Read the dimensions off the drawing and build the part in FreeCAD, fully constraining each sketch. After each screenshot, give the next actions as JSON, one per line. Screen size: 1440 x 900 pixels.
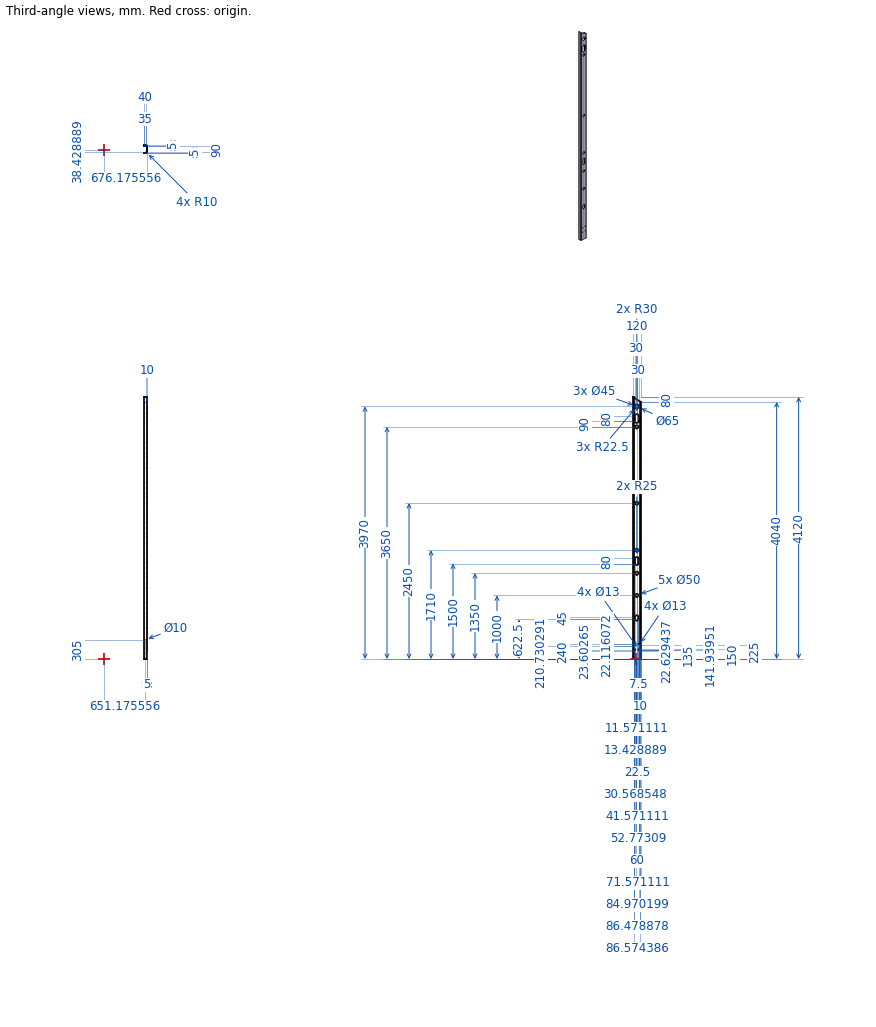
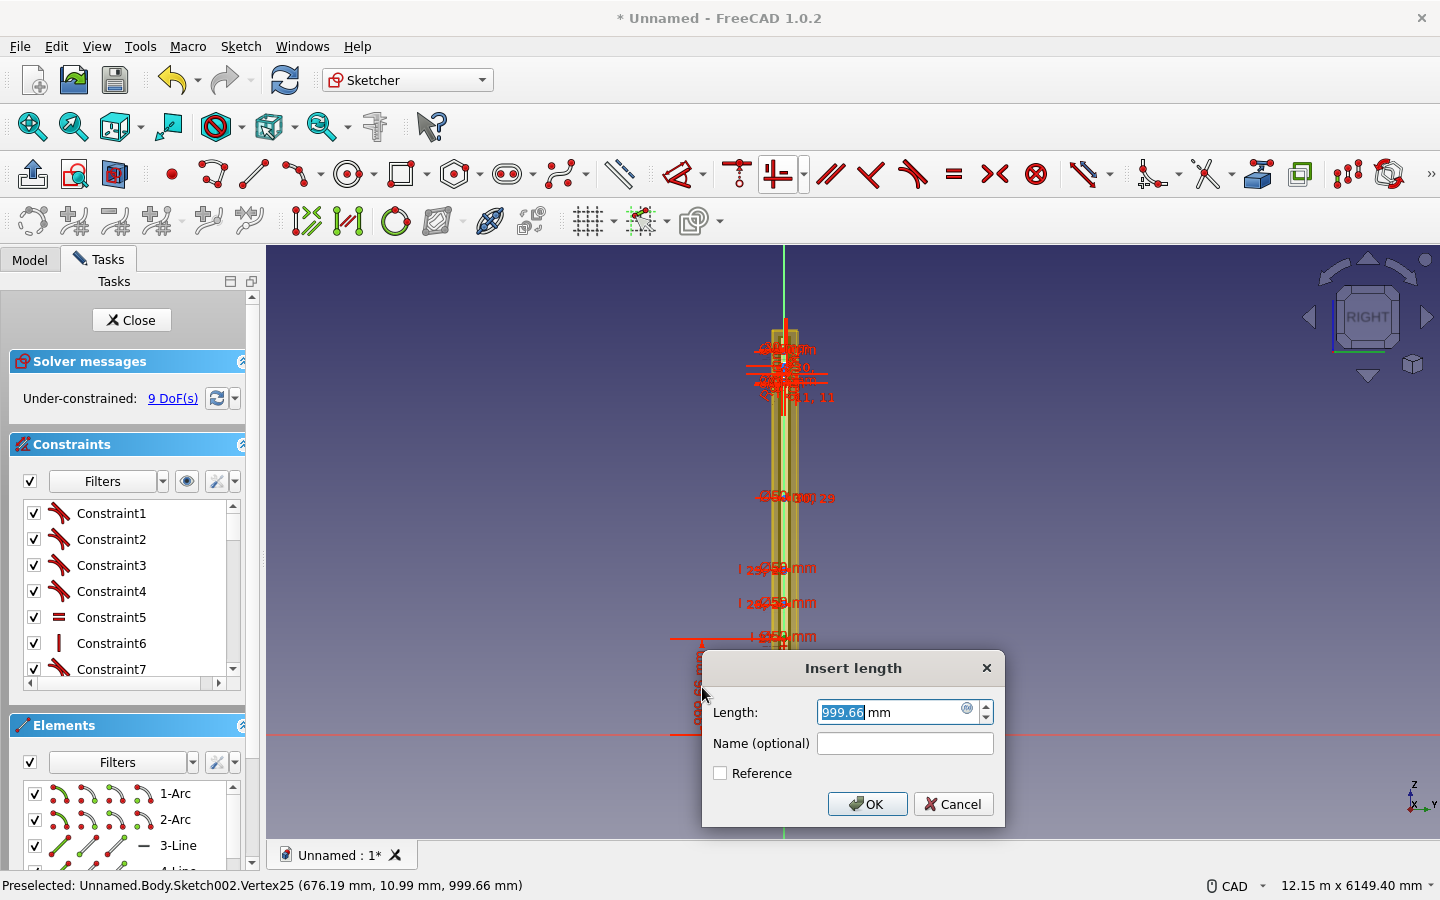
{"action": "type", "text": "1000"}
{"action": "key", "text": "Return"}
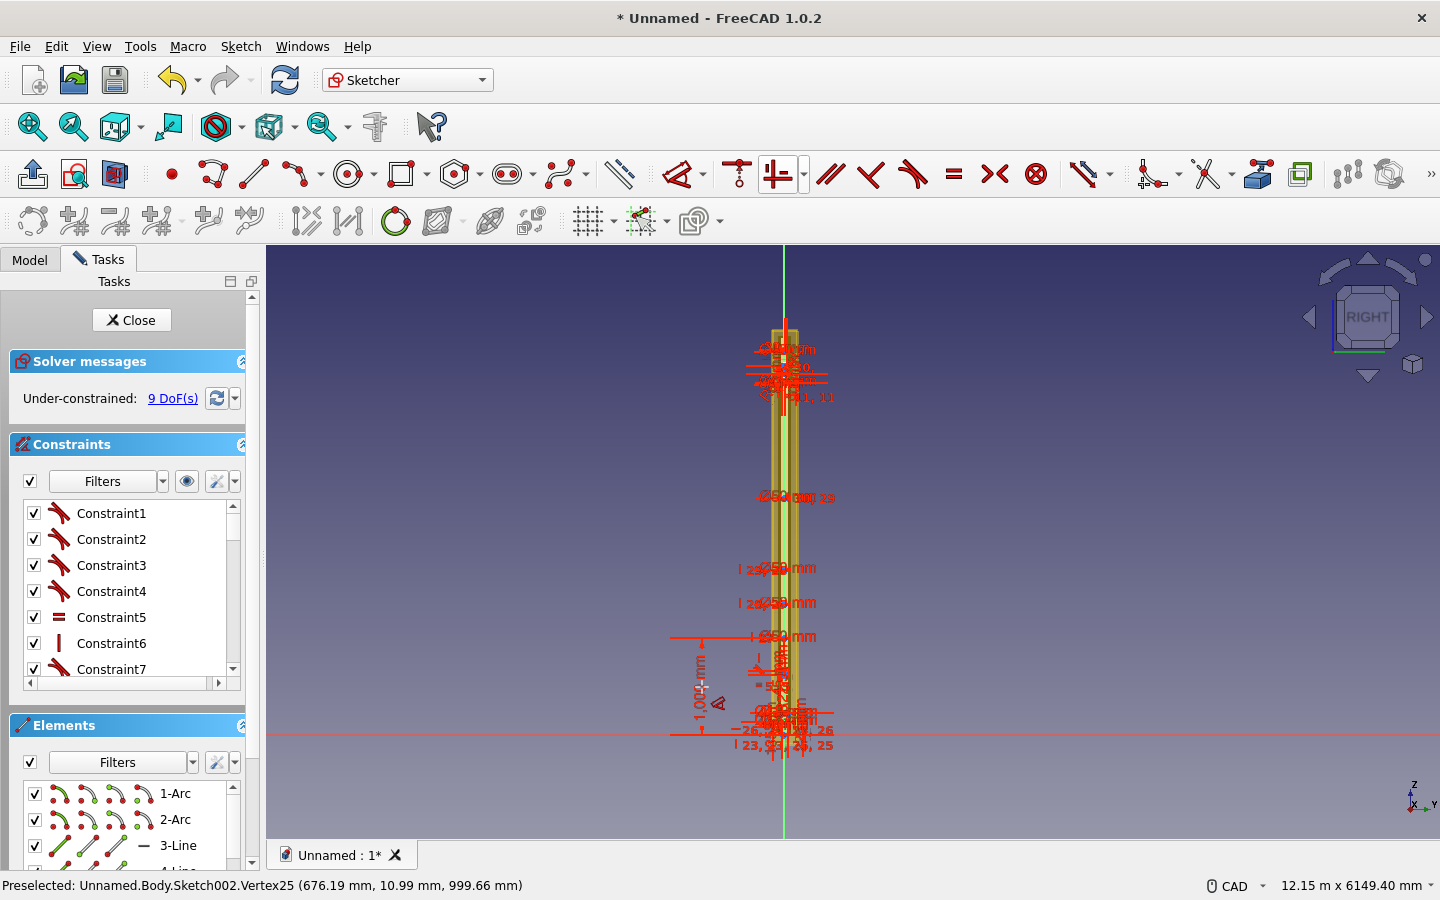
{"action": "left_click", "coordinate": [785, 605]}
{"action": "left_click", "coordinate": [750, 640]}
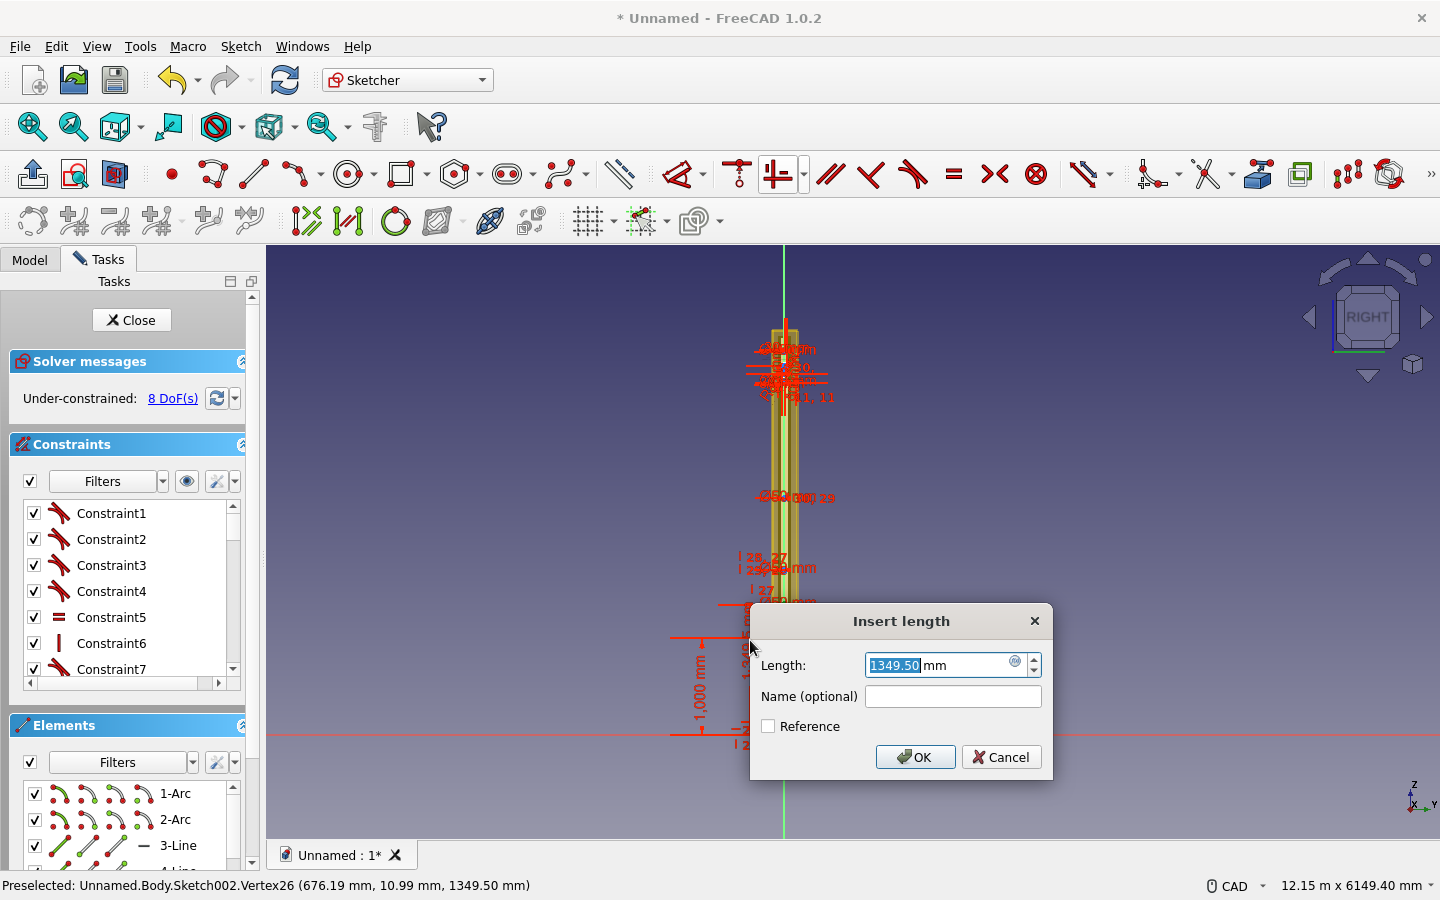
{"action": "type", "text": "1350"}
{"action": "key", "text": "Return"}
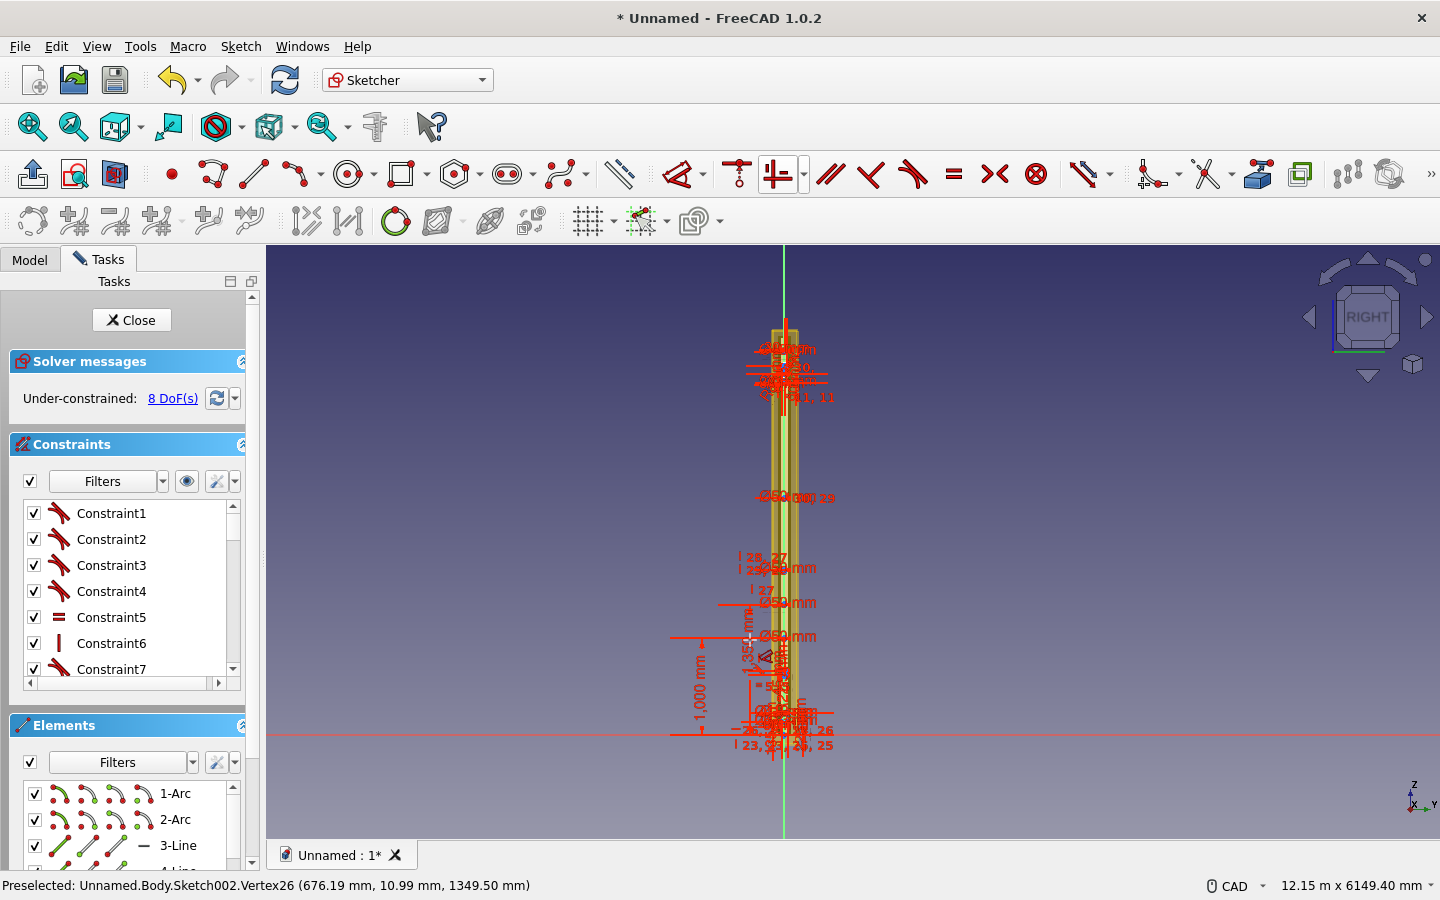
{"action": "left_click", "coordinate": [785, 352]}
{"action": "left_click", "coordinate": [750, 543]}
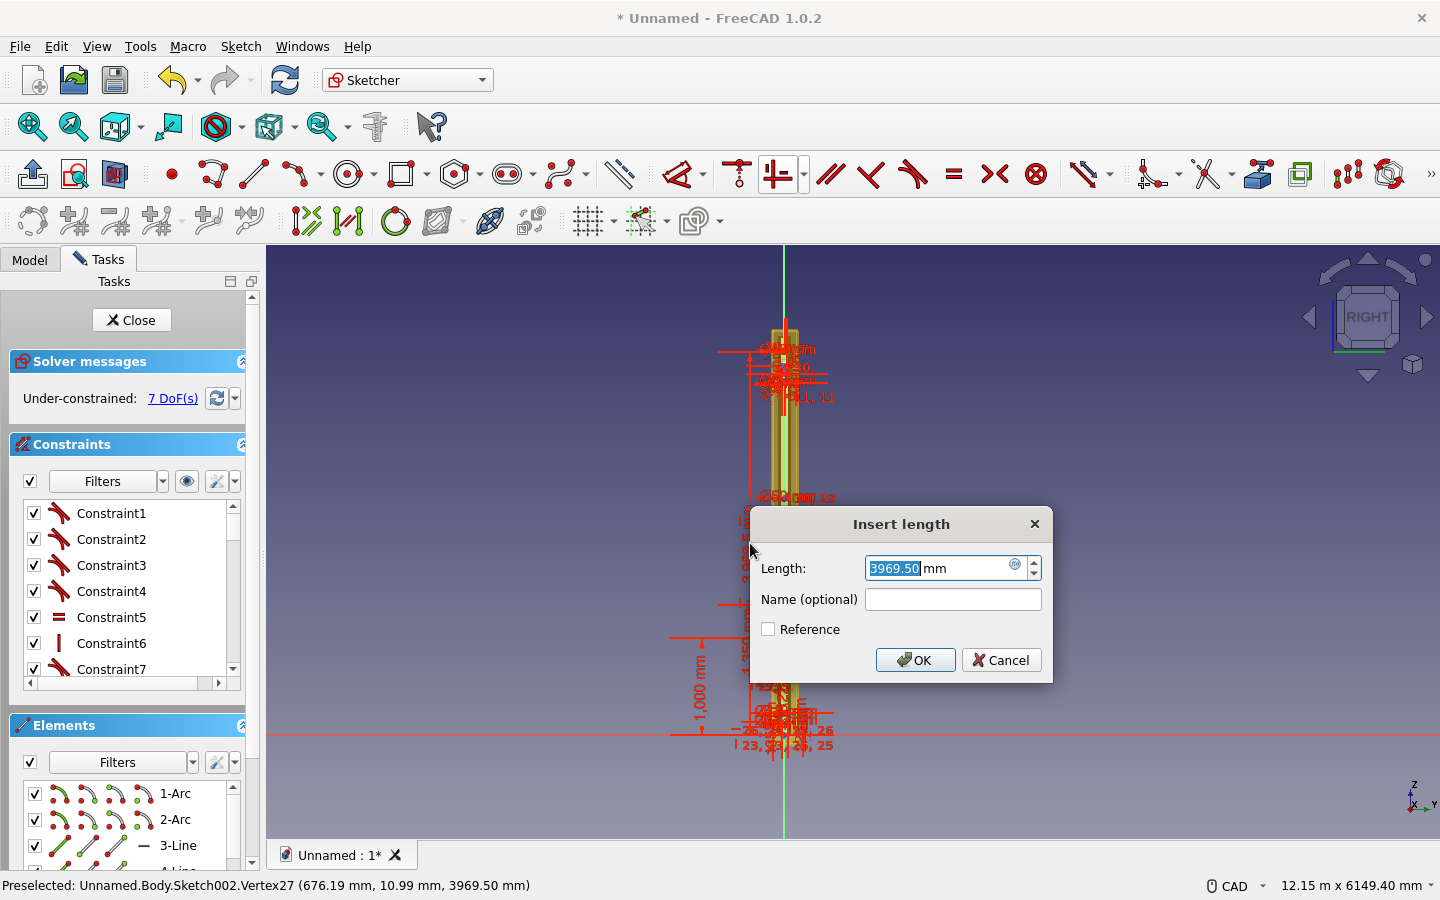
{"action": "type", "text": "3970"}
{"action": "key", "text": "Return"}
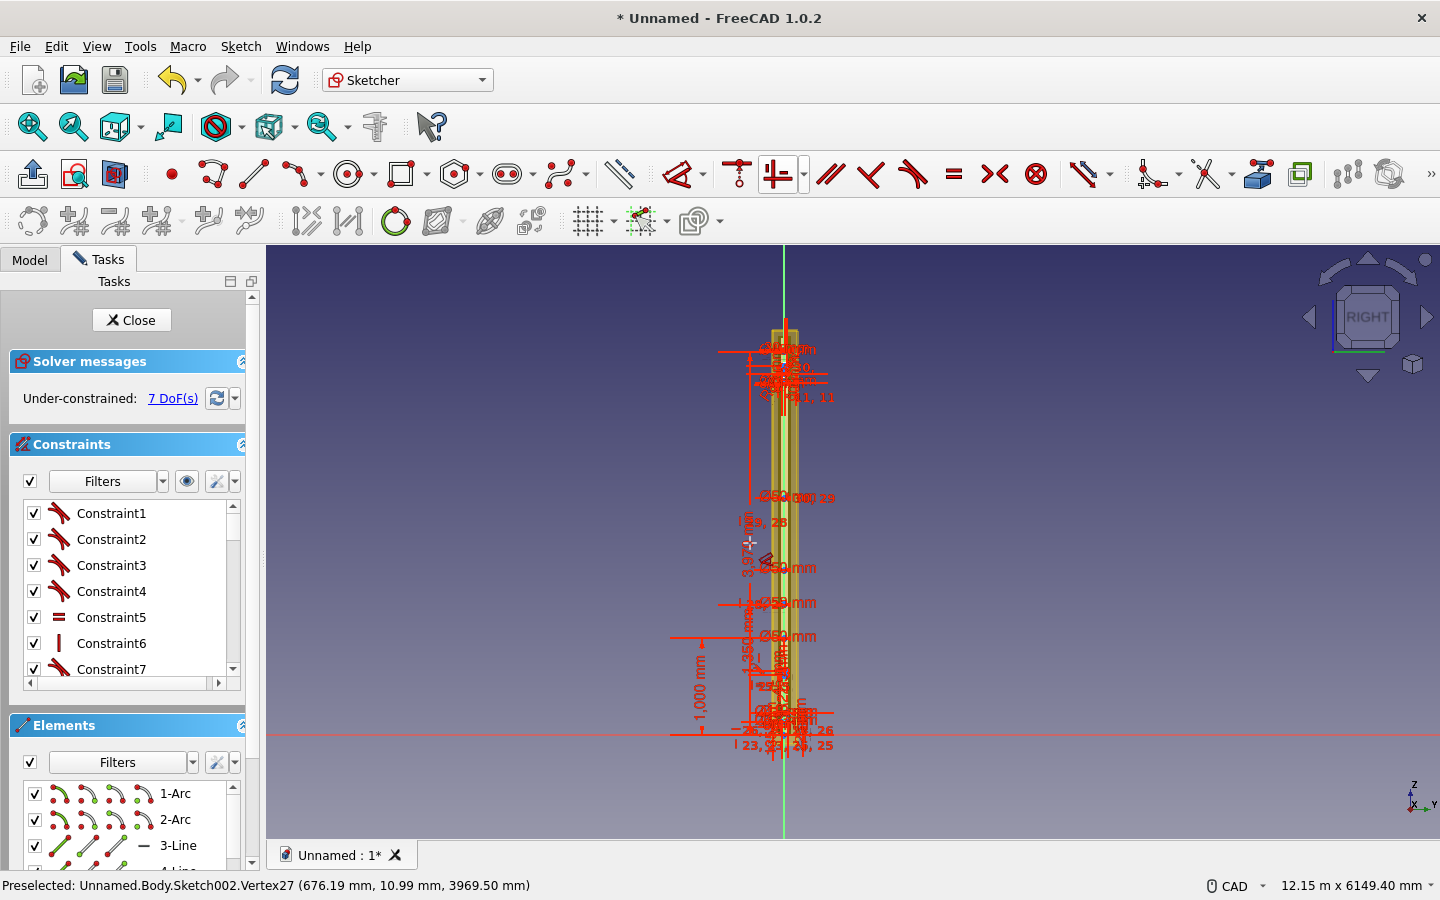
{"action": "scroll", "coordinate": [785, 383], "scroll_direction": "up", "scroll_amount": 2}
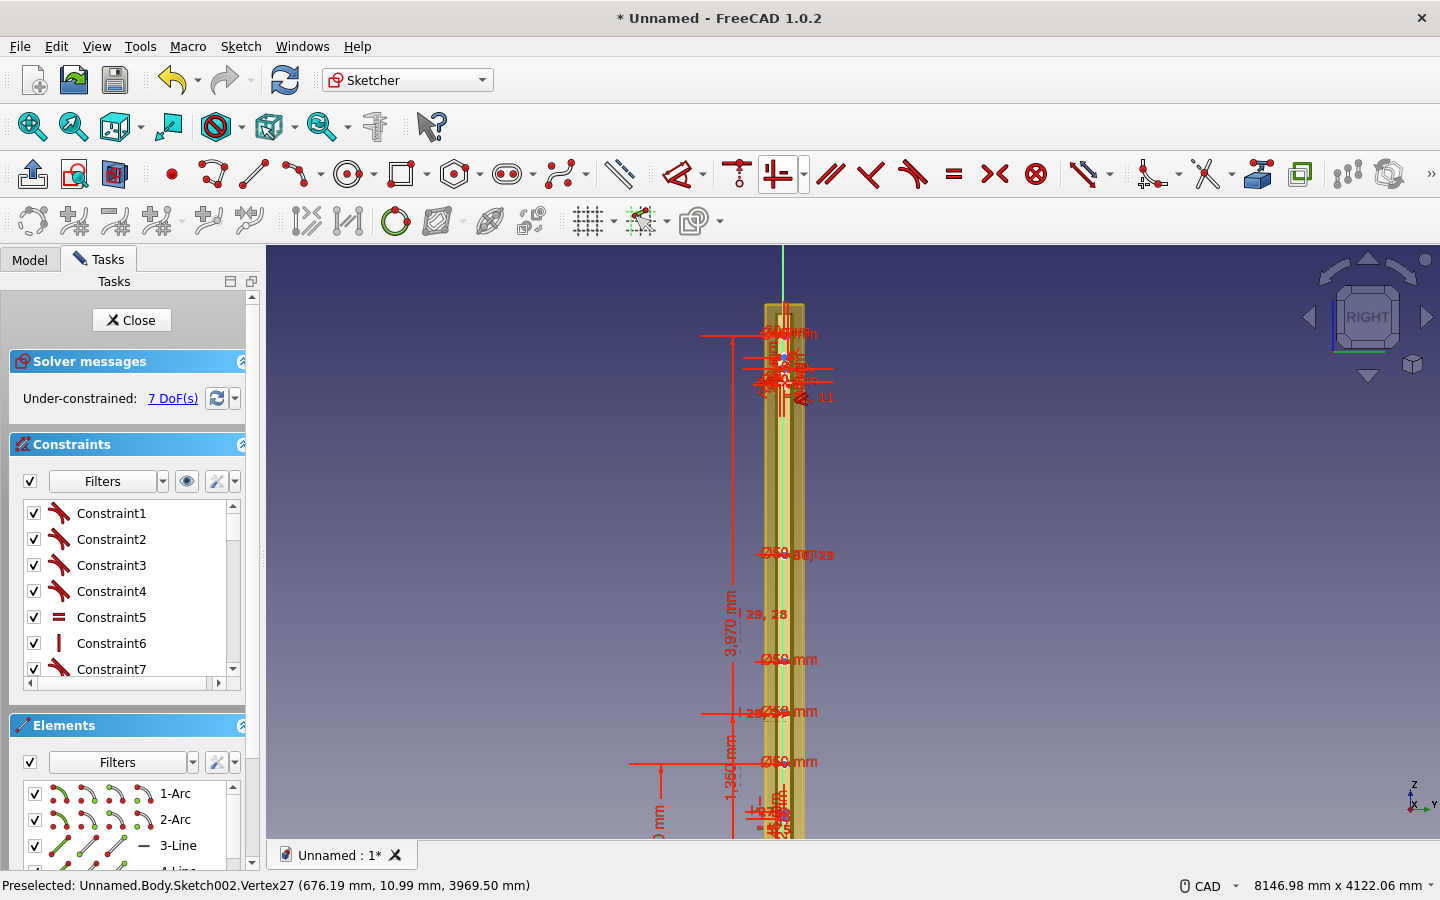
{"action": "left_click", "coordinate": [784, 382]}
{"action": "left_click", "coordinate": [749, 597]}